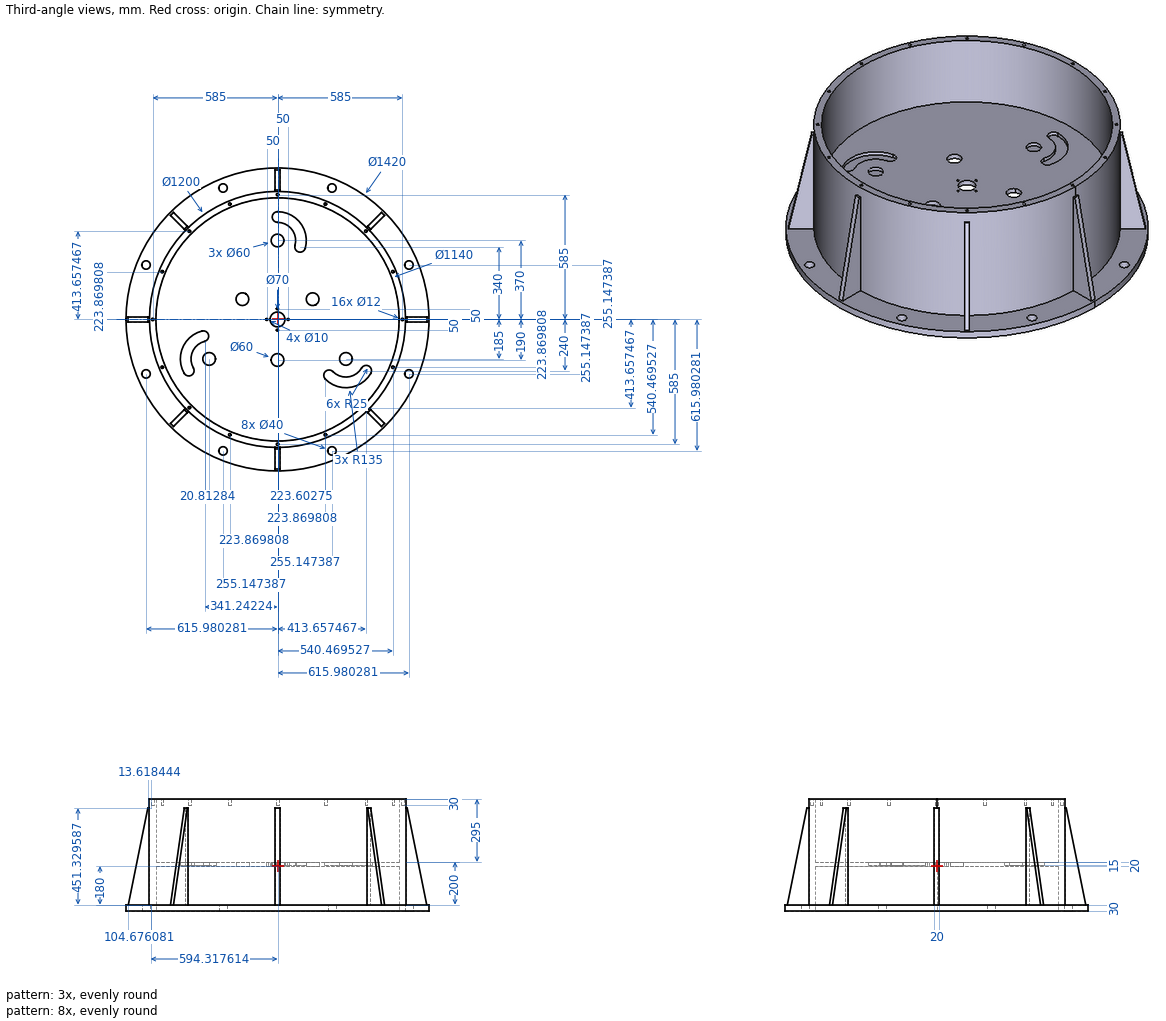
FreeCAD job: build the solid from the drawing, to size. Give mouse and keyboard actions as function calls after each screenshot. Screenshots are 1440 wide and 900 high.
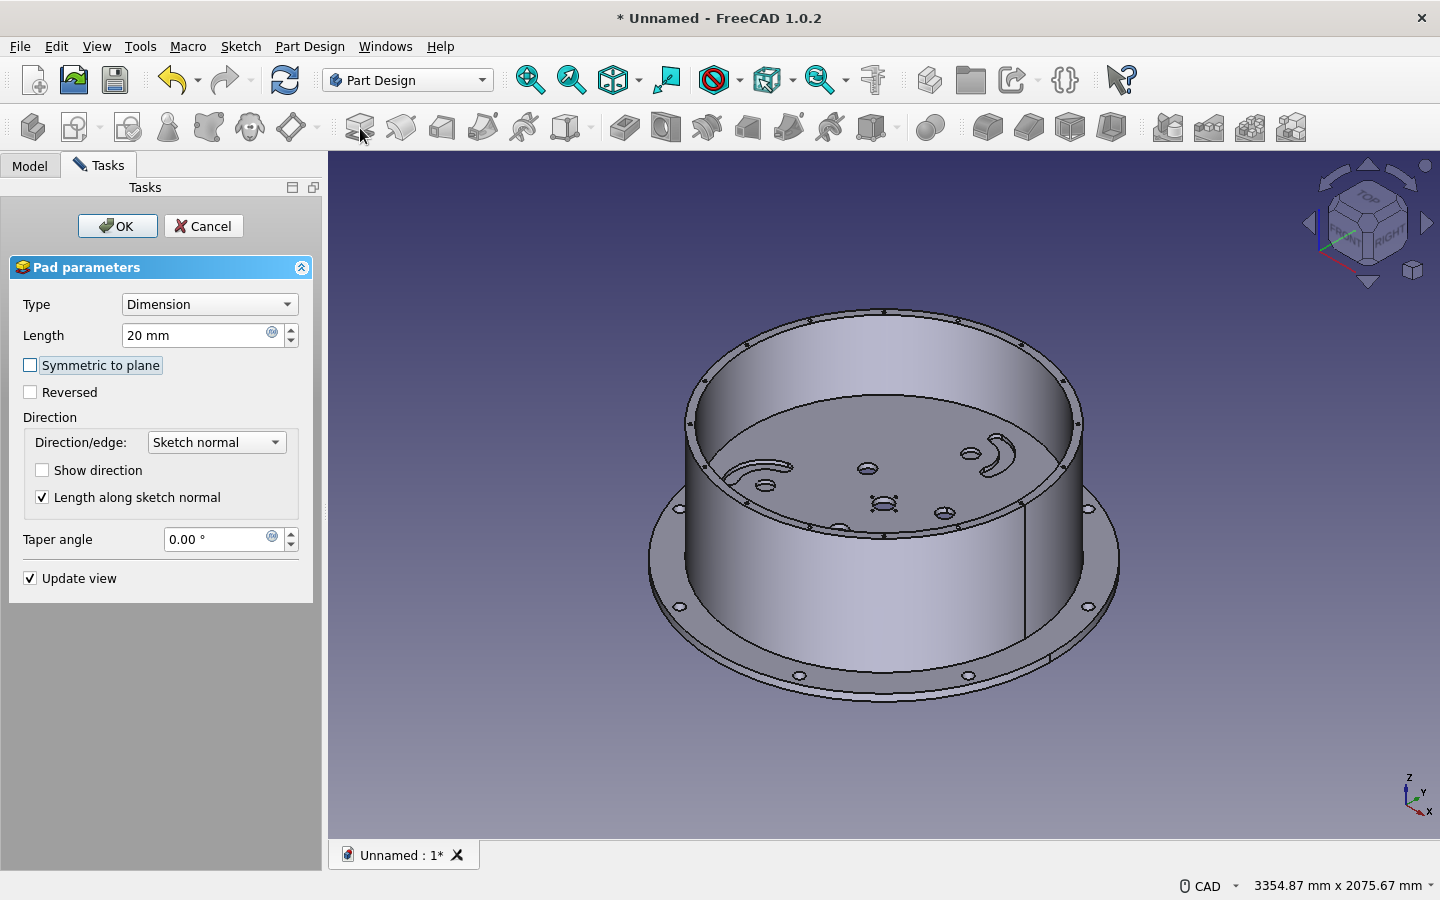
click(31, 365)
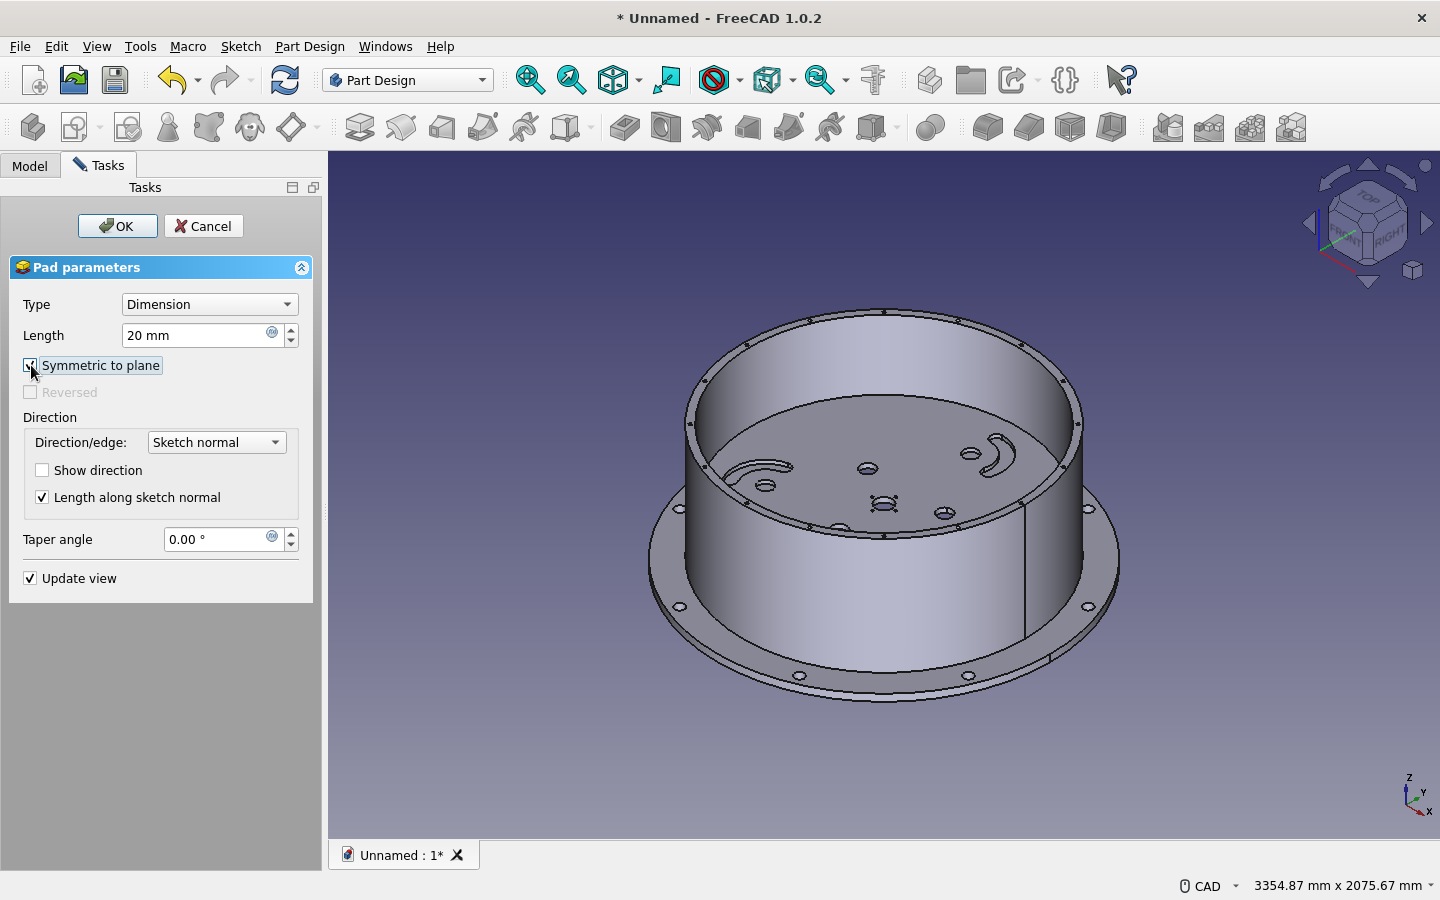
click(118, 226)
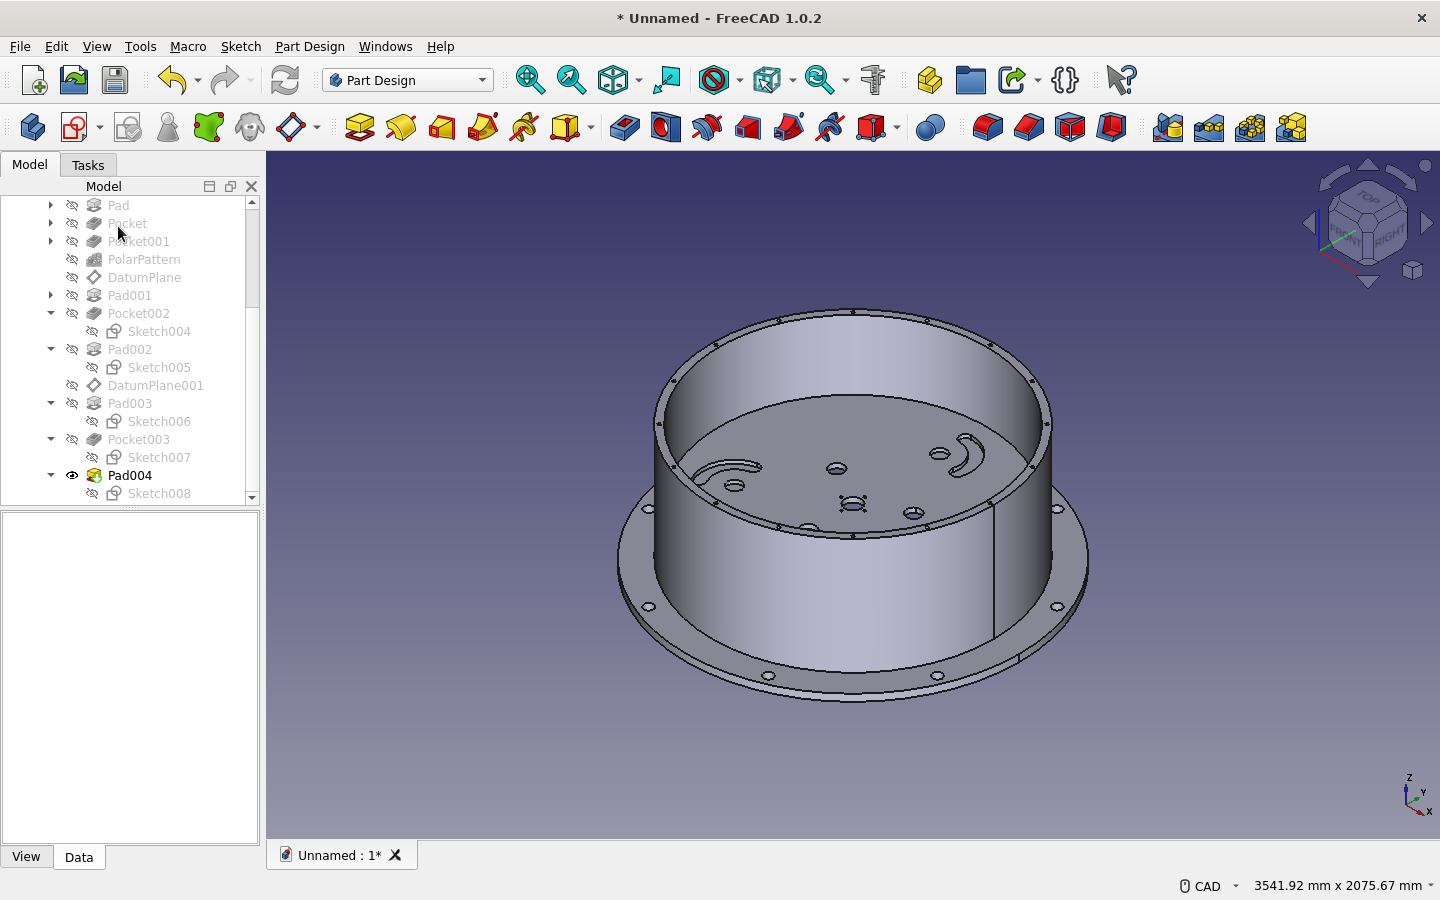
click(117, 475)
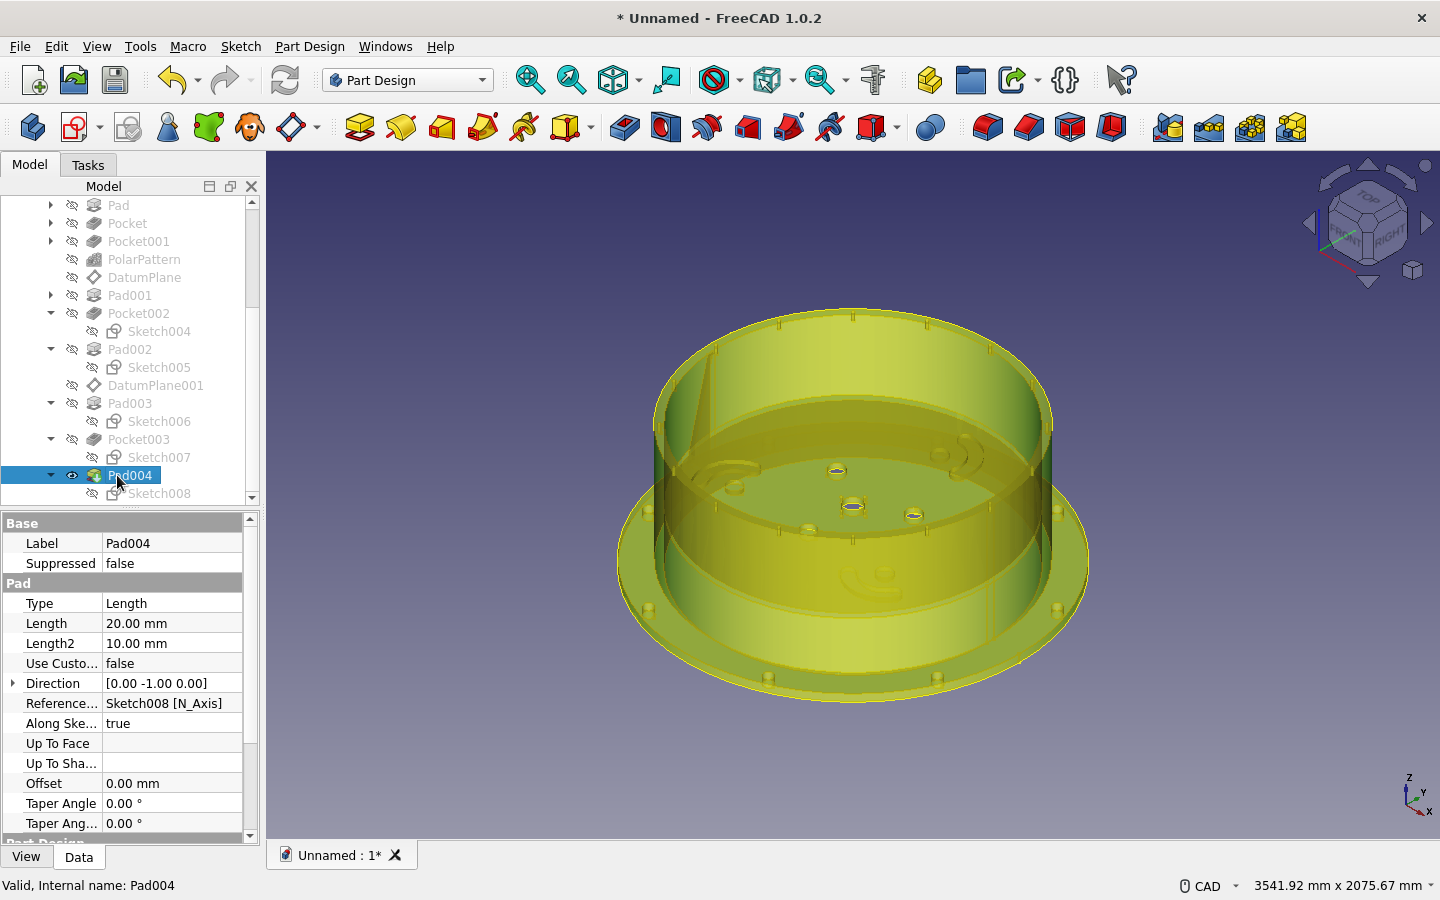
click(1250, 128)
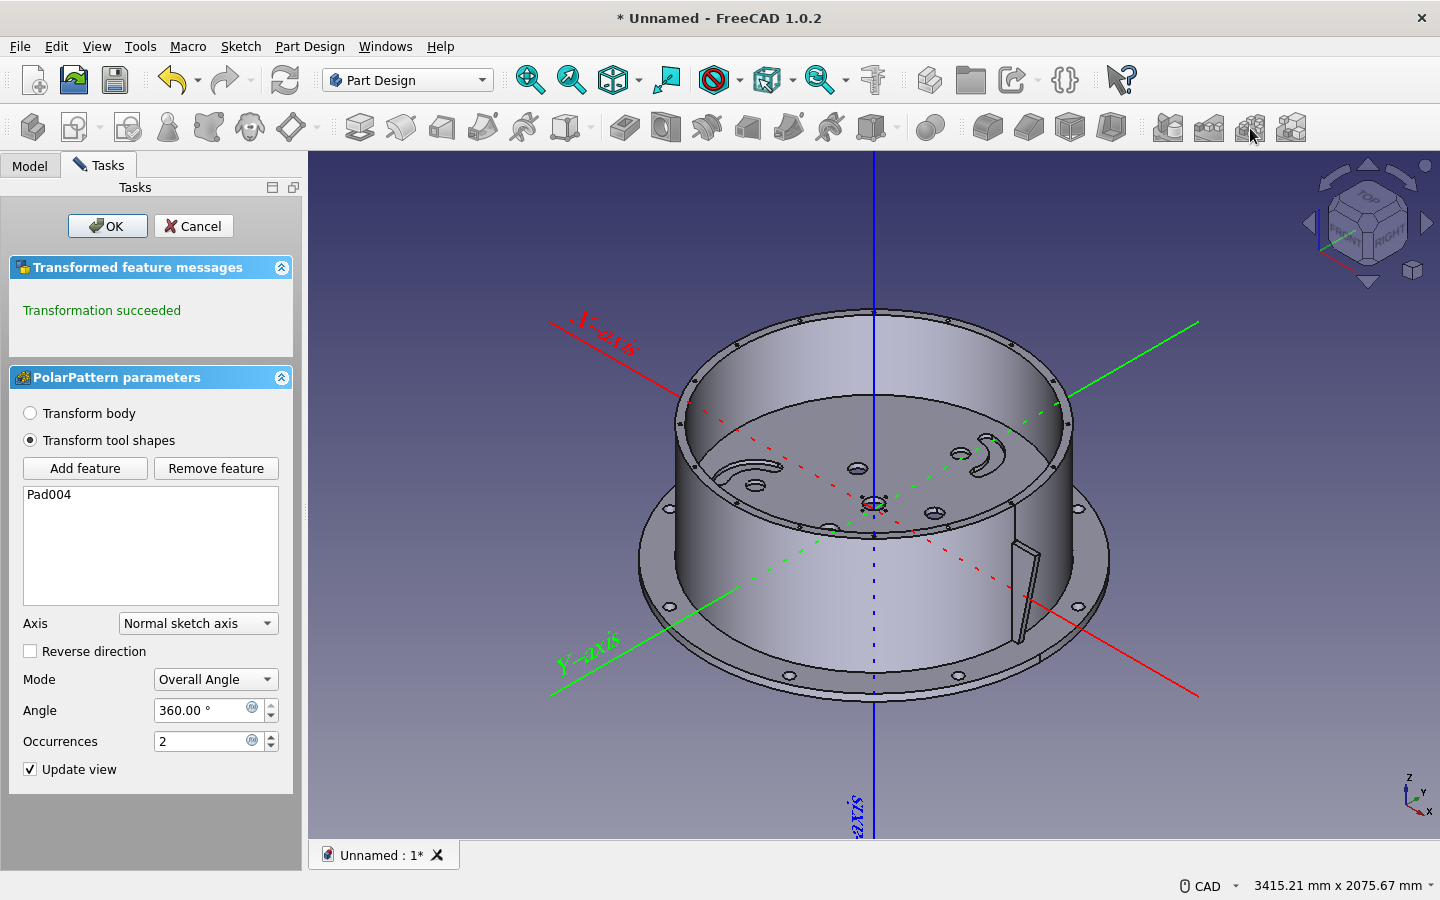
click(199, 624)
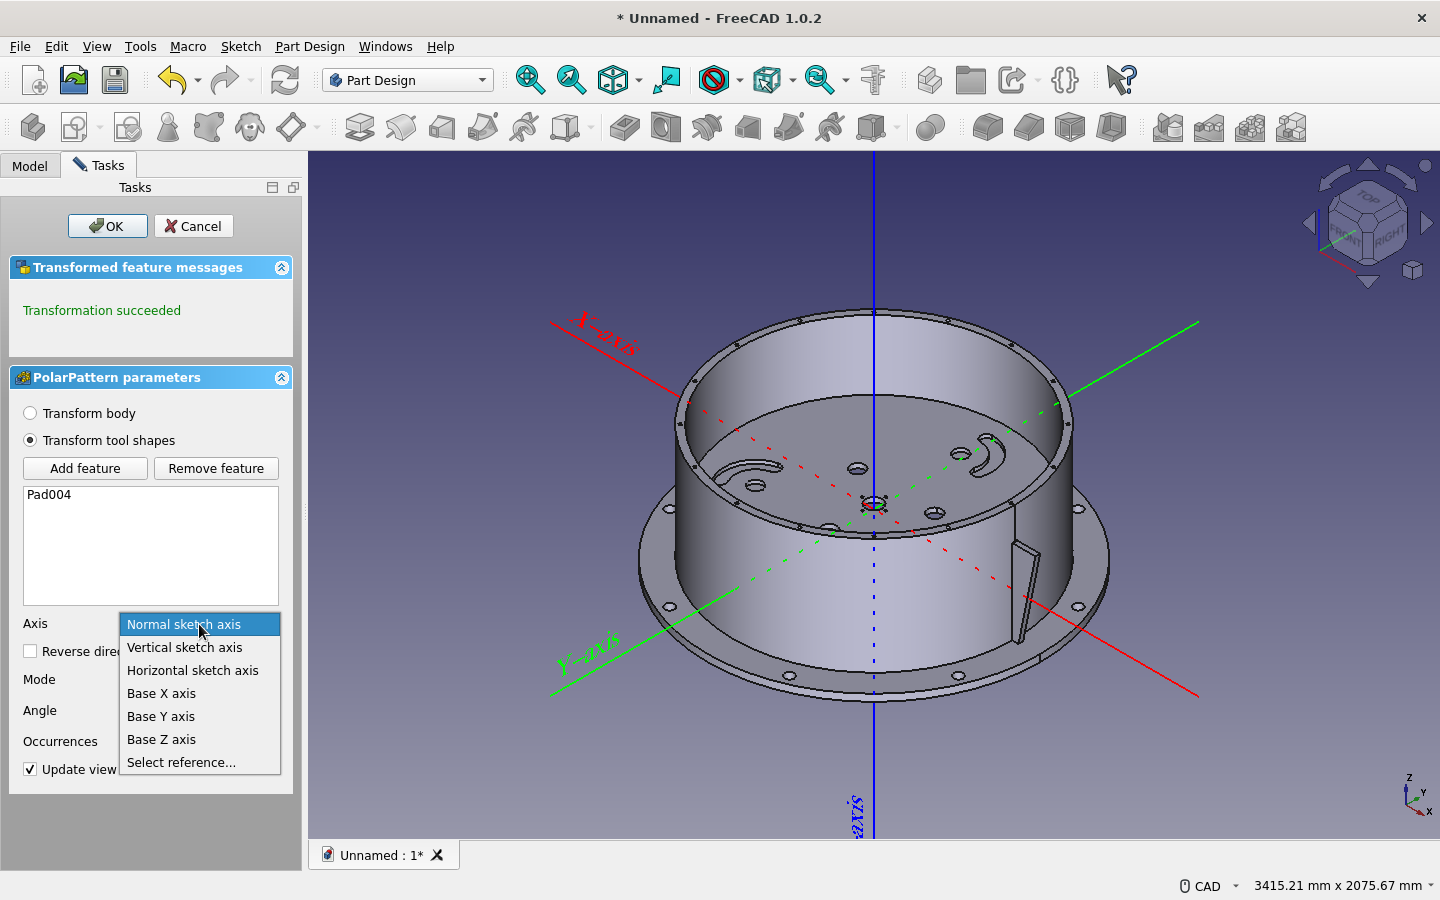
click(198, 740)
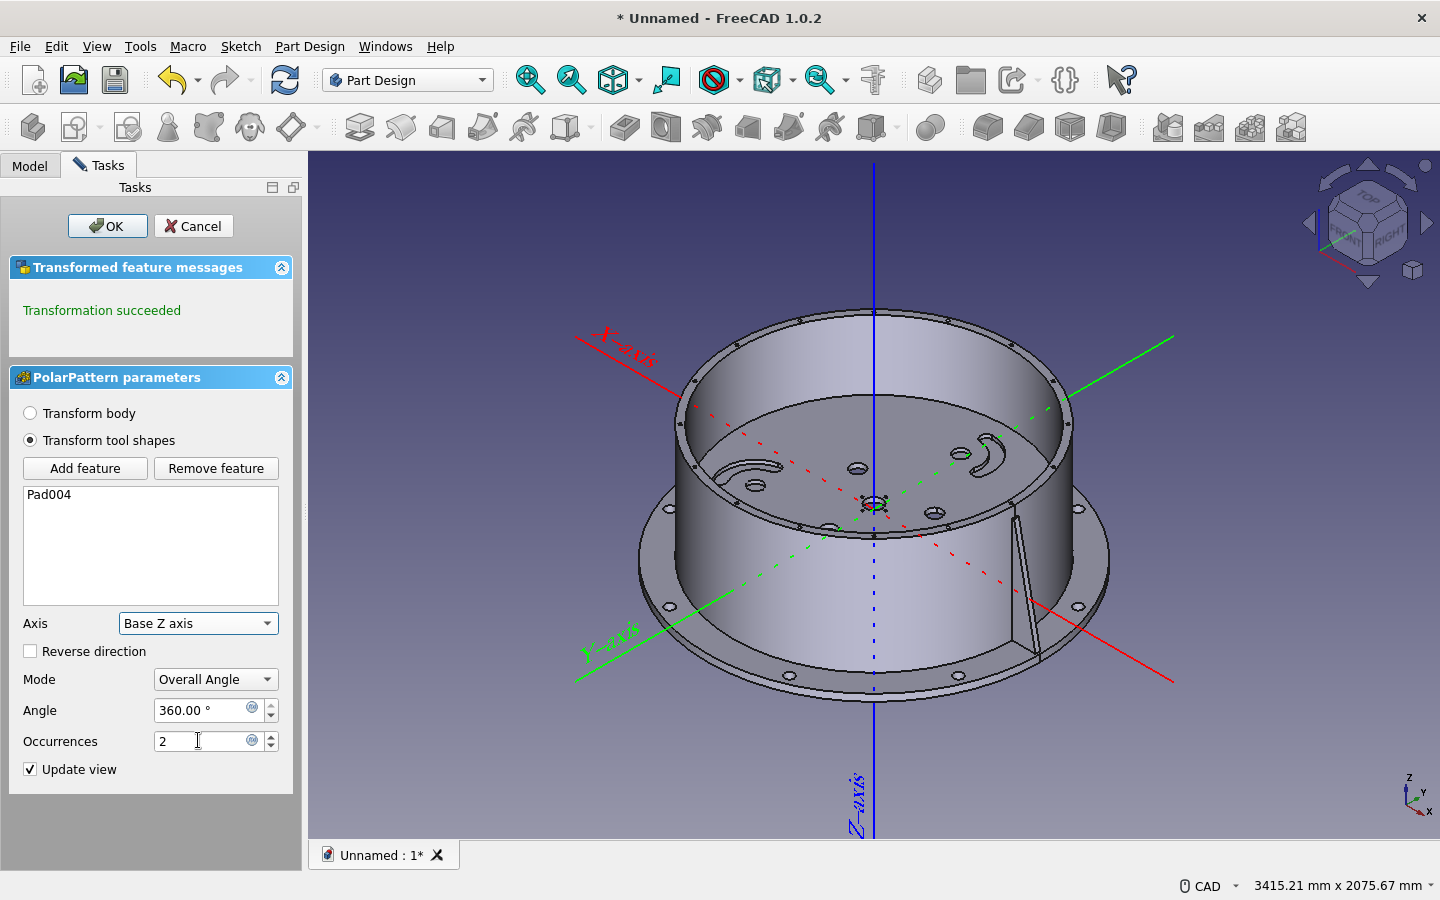
triple_click(210, 742)